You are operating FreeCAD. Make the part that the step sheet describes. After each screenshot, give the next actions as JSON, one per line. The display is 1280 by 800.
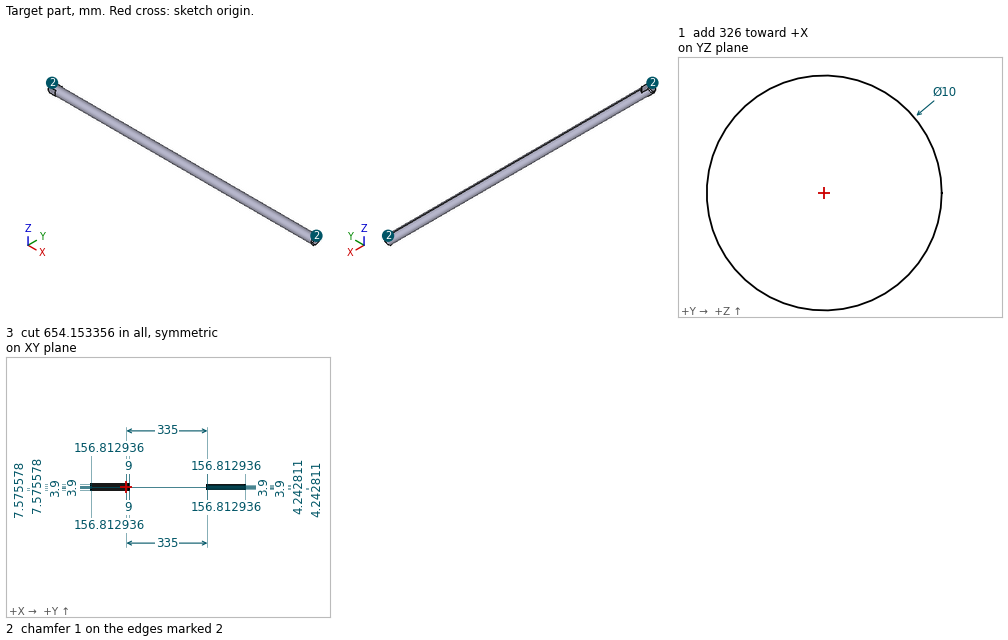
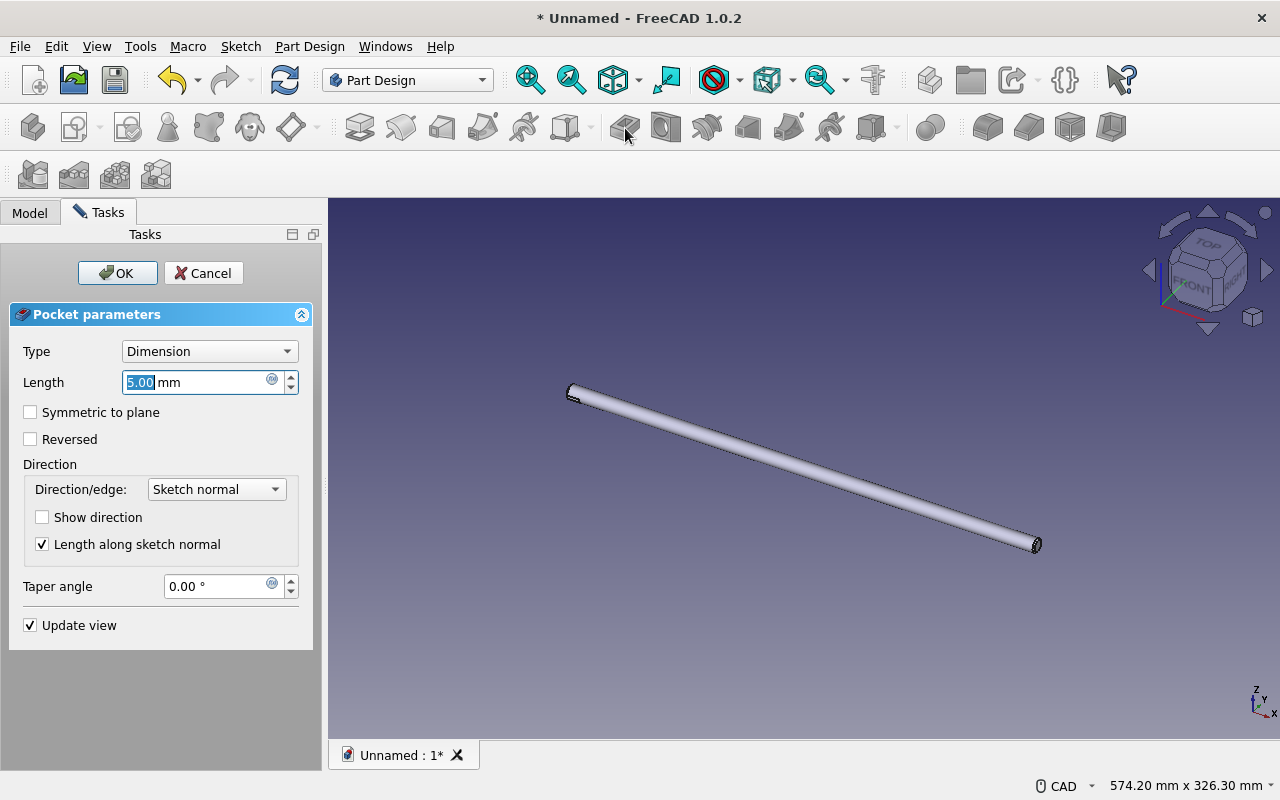
{"action": "type", "text": "654.153356"}
{"action": "key", "text": "Tab"}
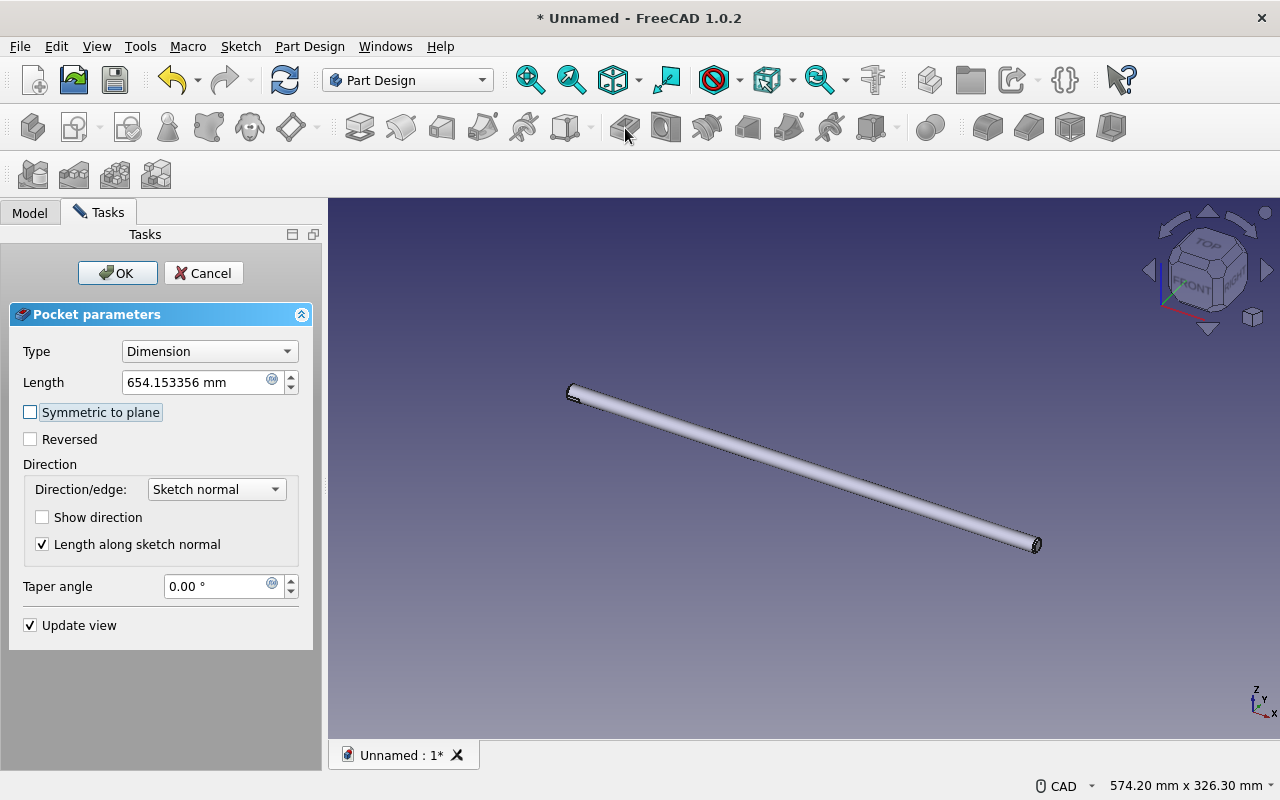
{"action": "left_click", "coordinate": [31, 412]}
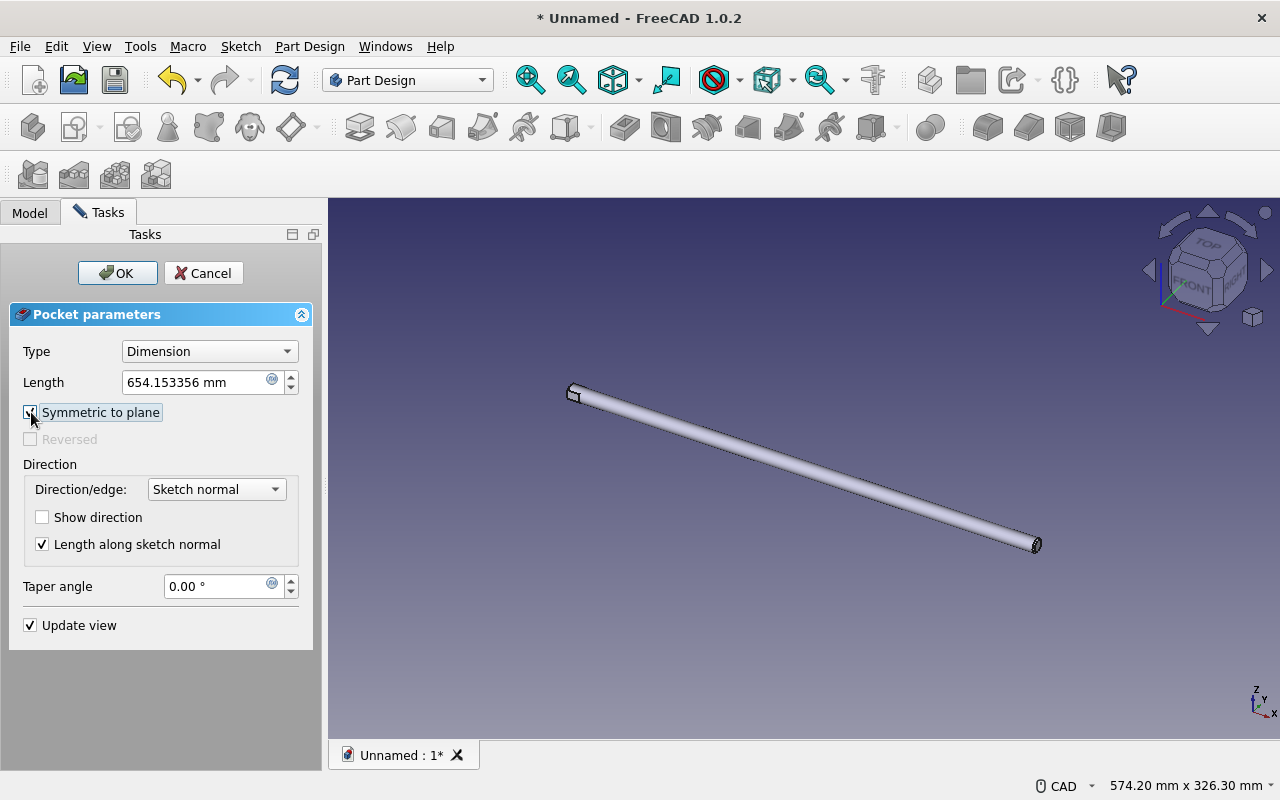
{"action": "left_click", "coordinate": [118, 273]}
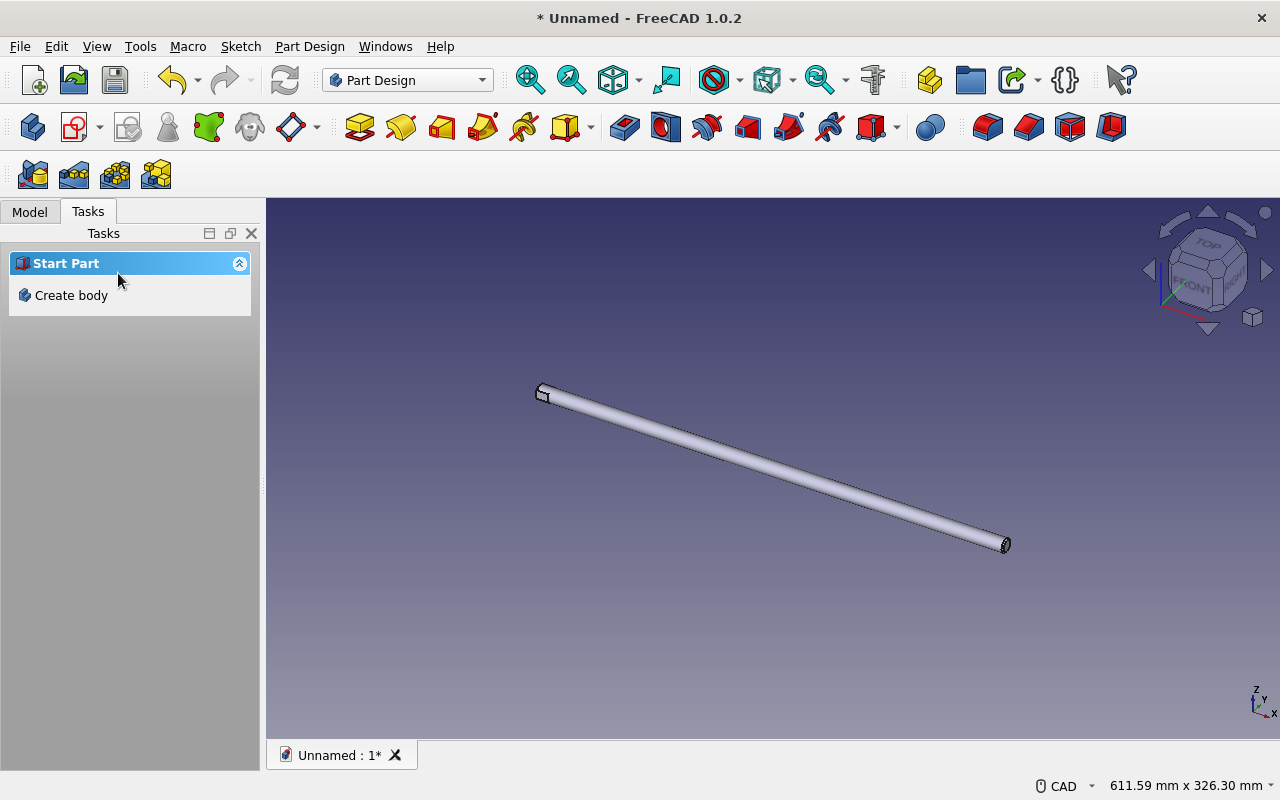
{"action": "key", "text": "0"}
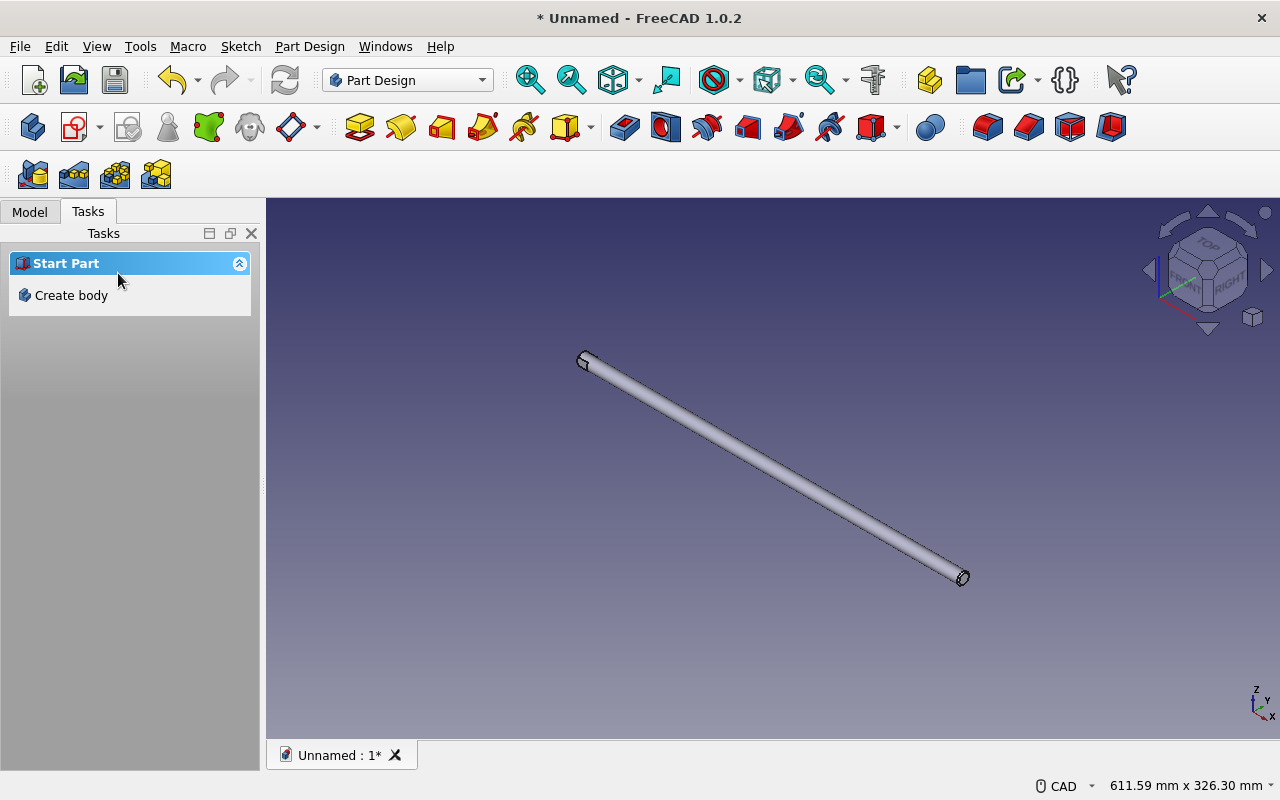
{"action": "key", "text": "v f"}